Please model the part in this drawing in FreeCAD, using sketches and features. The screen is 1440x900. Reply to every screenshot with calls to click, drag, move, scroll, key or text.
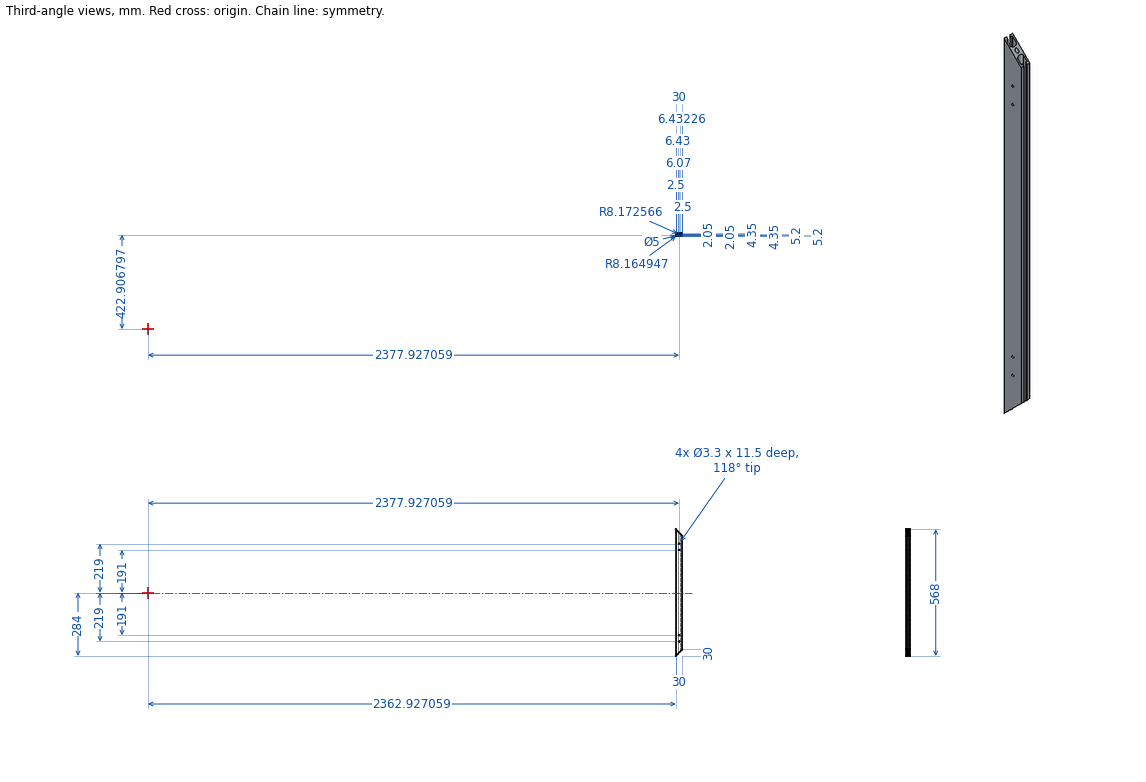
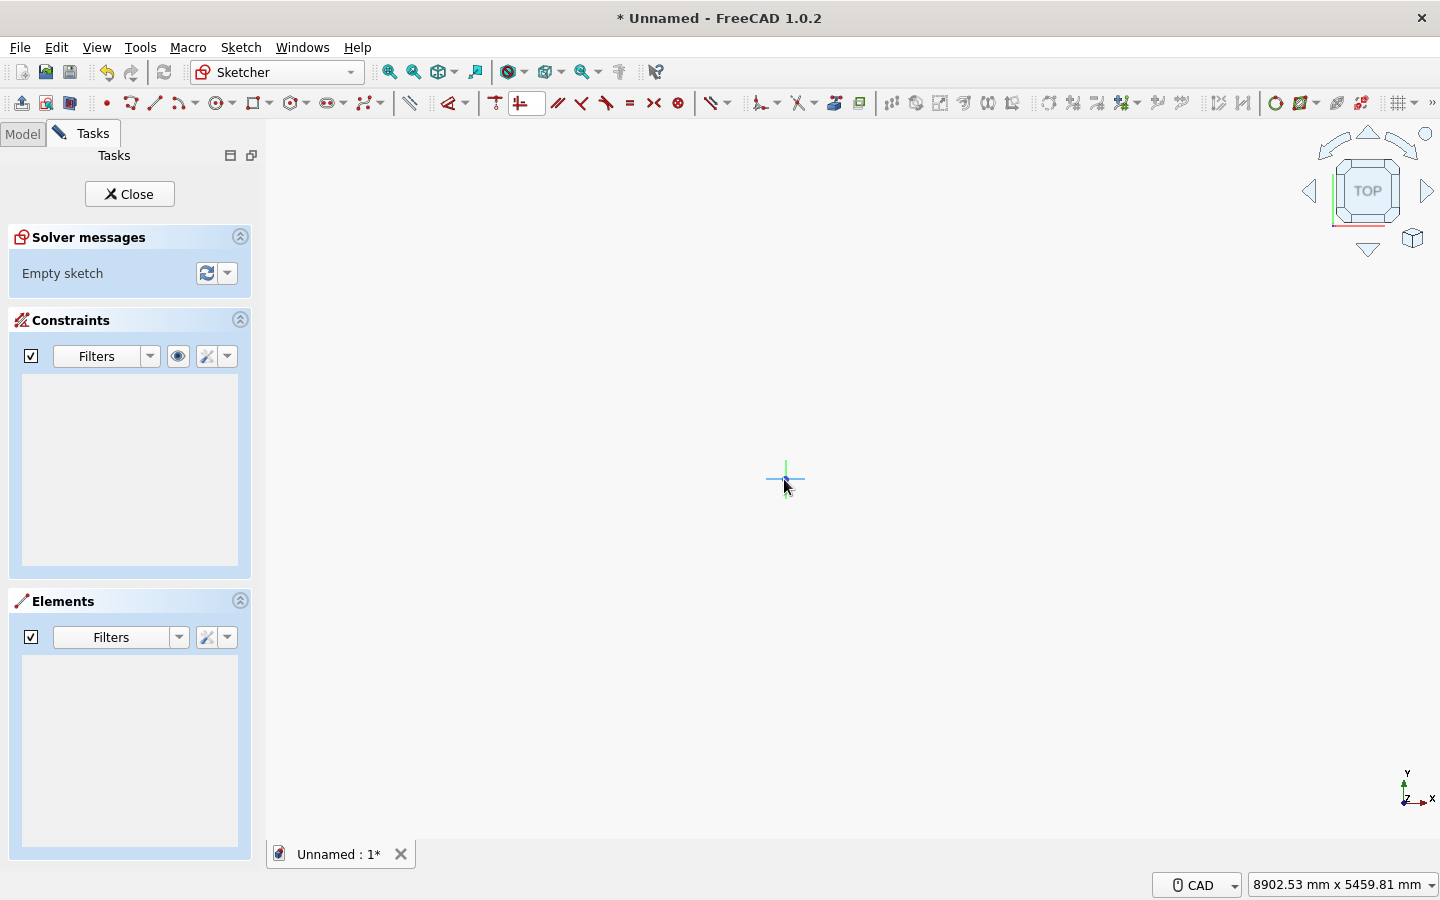
scroll(1116, 421, up, 15)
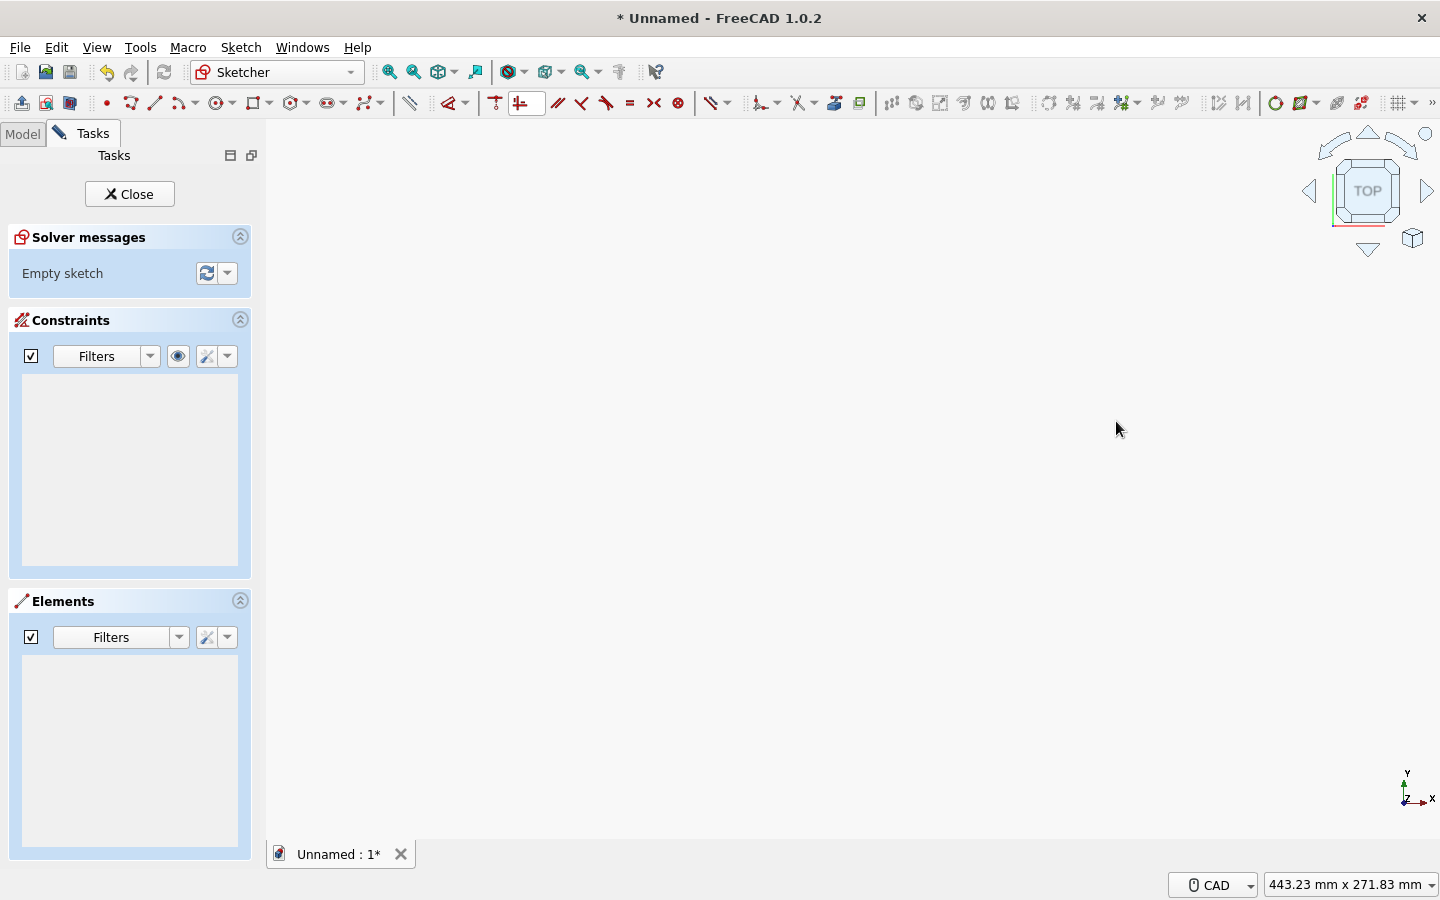
click(132, 104)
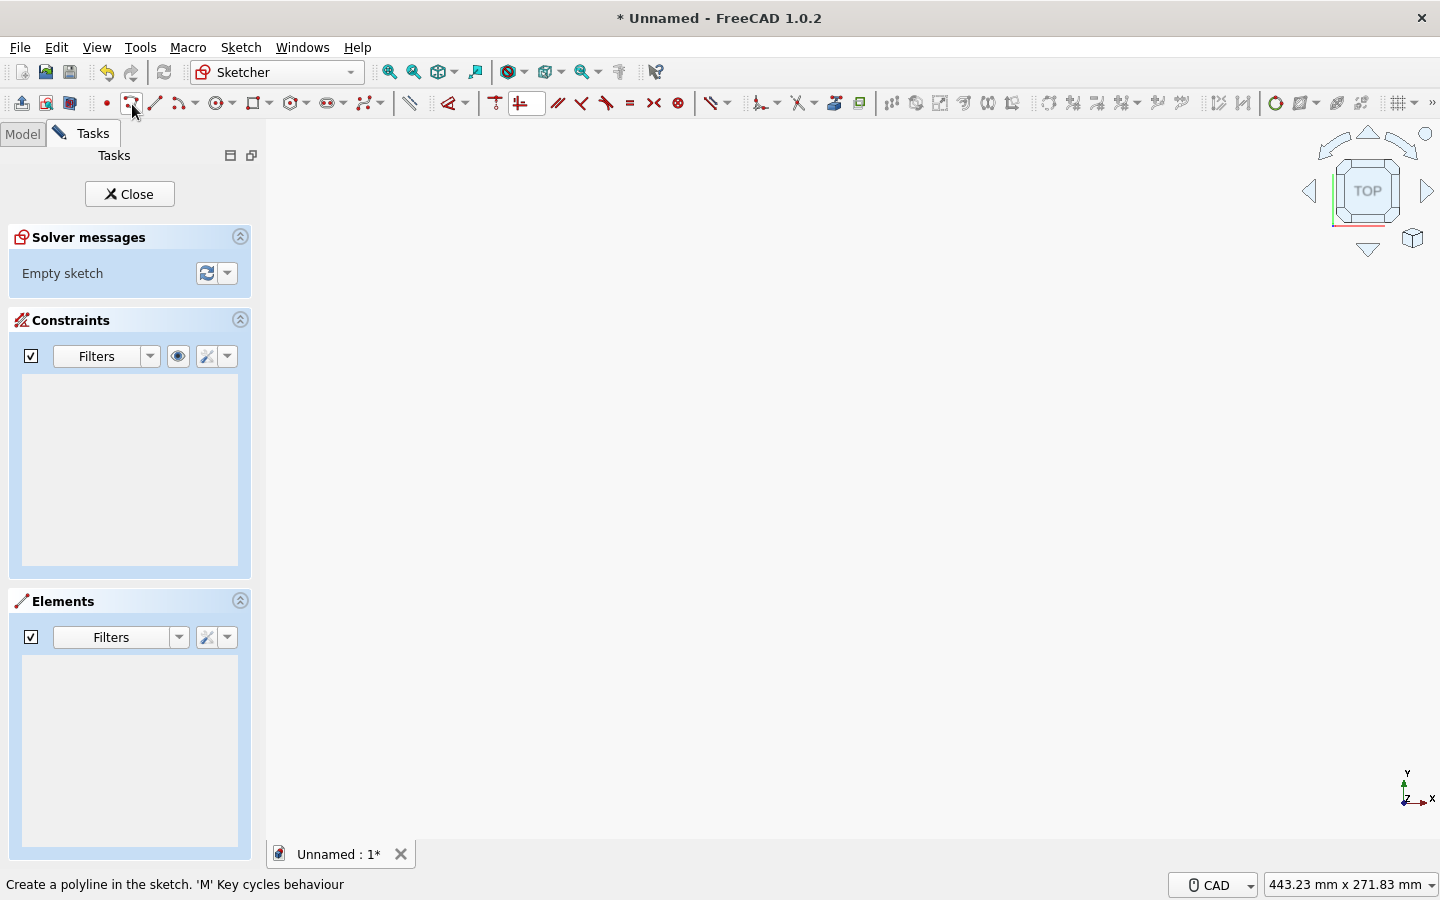
click(782, 454)
click(799, 454)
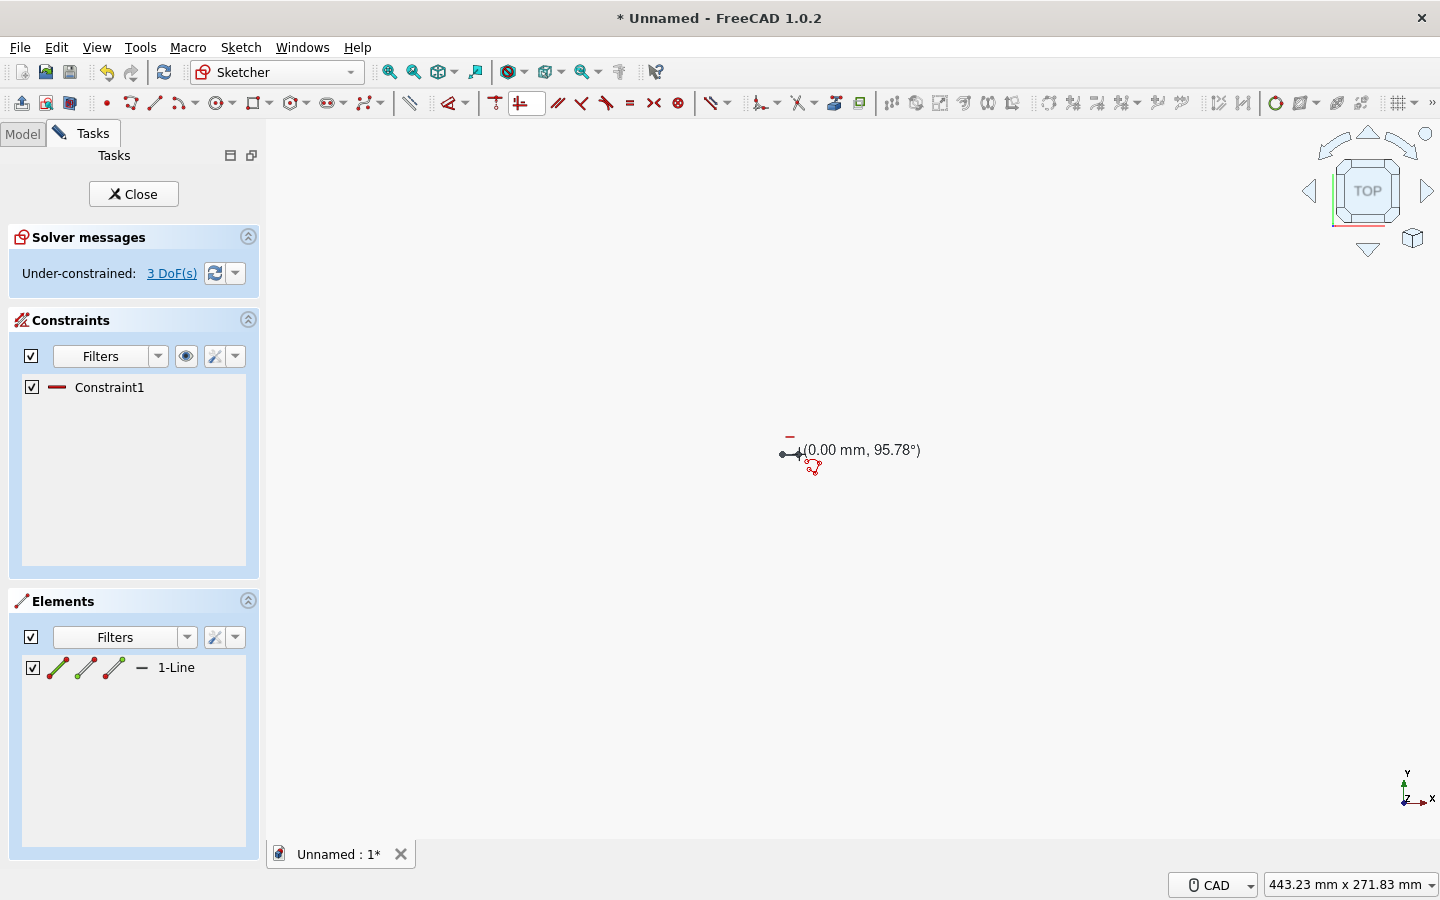
scroll(799, 459, up, 6)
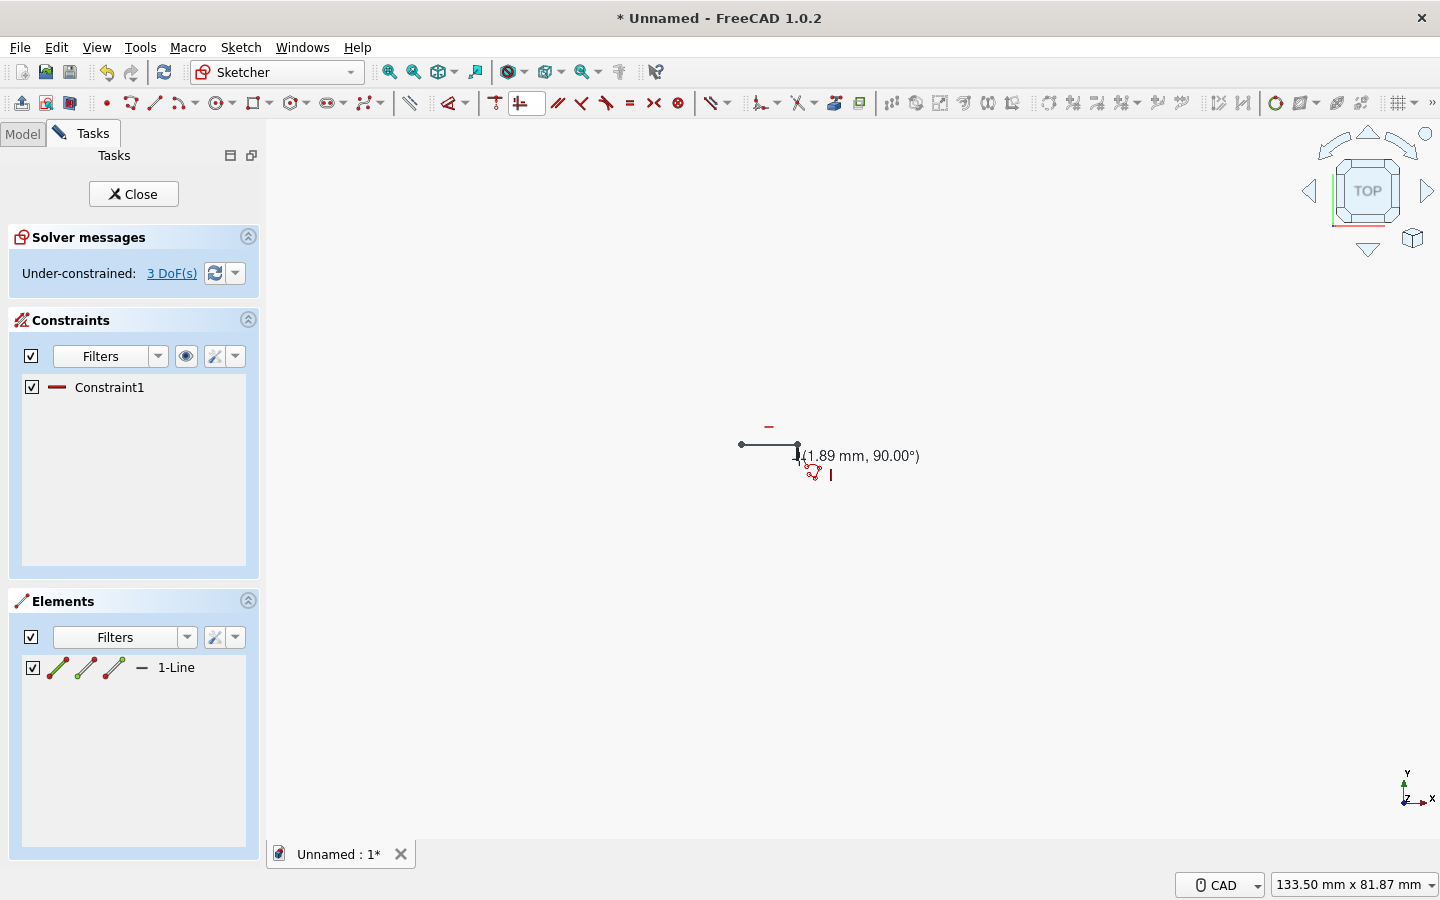
click(798, 459)
click(821, 459)
click(821, 421)
click(558, 421)
click(558, 459)
click(580, 459)
click(580, 441)
click(636, 441)
right_click(636, 441)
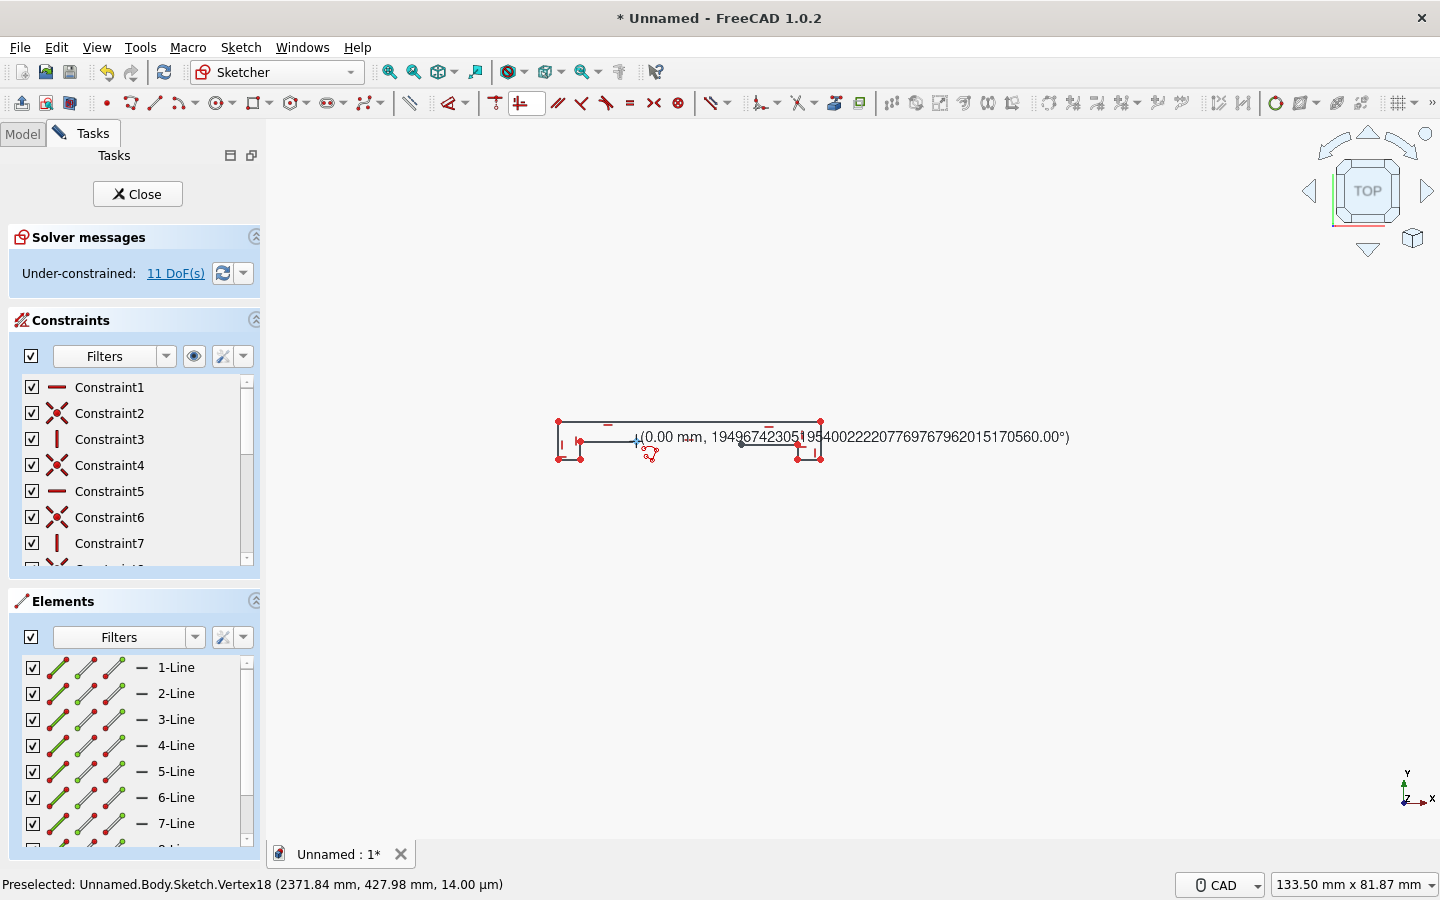
click(636, 532)
click(580, 532)
click(580, 514)
click(558, 514)
click(558, 553)
click(821, 553)
click(821, 514)
click(799, 514)
click(799, 532)
click(743, 532)
right_click(743, 532)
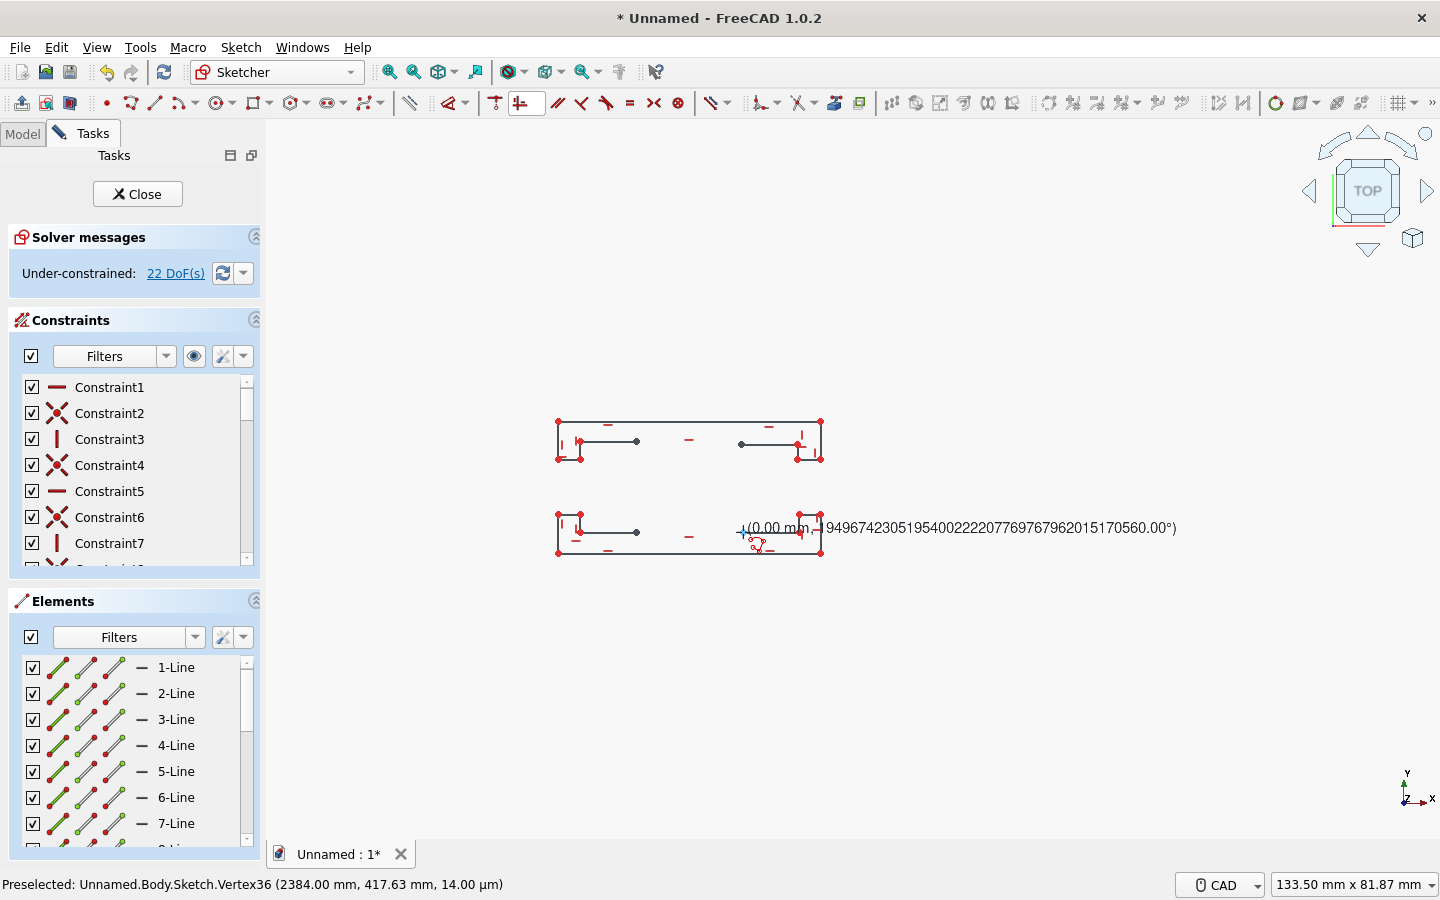
key(g)
key(3)
key(a)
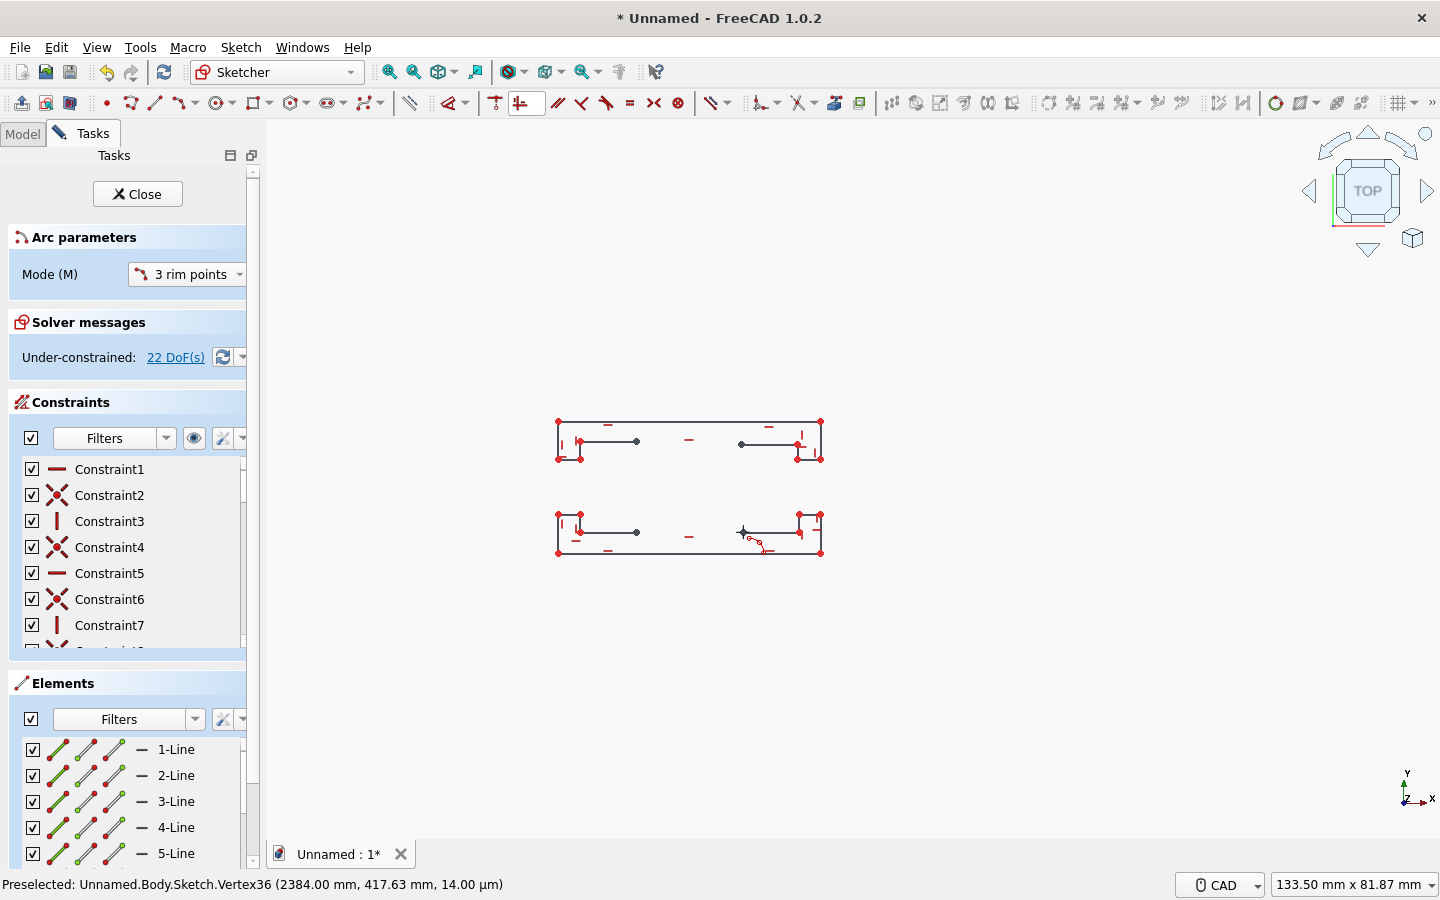
click(636, 442)
click(636, 533)
click(653, 487)